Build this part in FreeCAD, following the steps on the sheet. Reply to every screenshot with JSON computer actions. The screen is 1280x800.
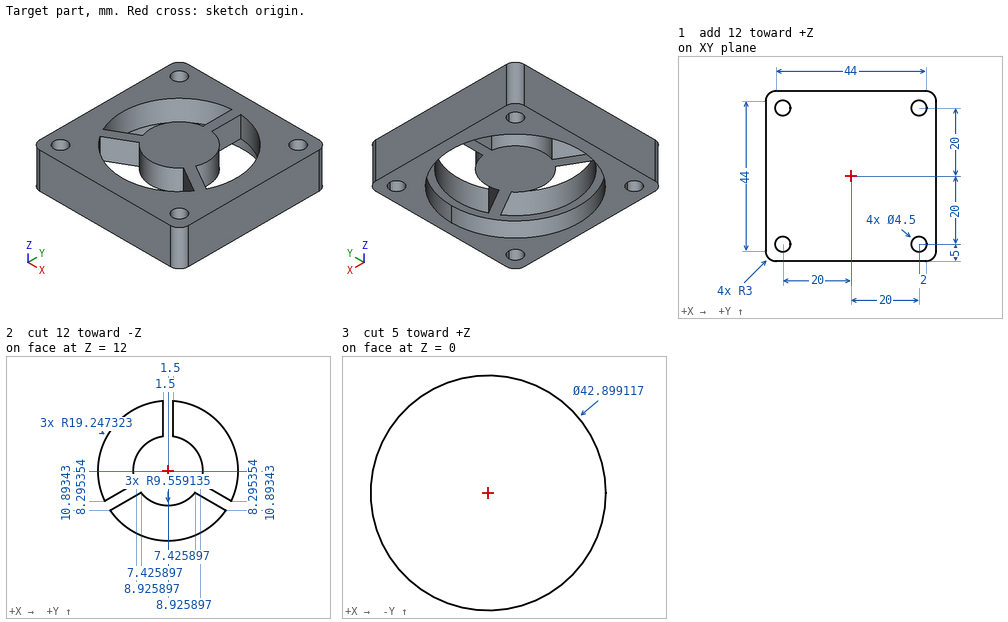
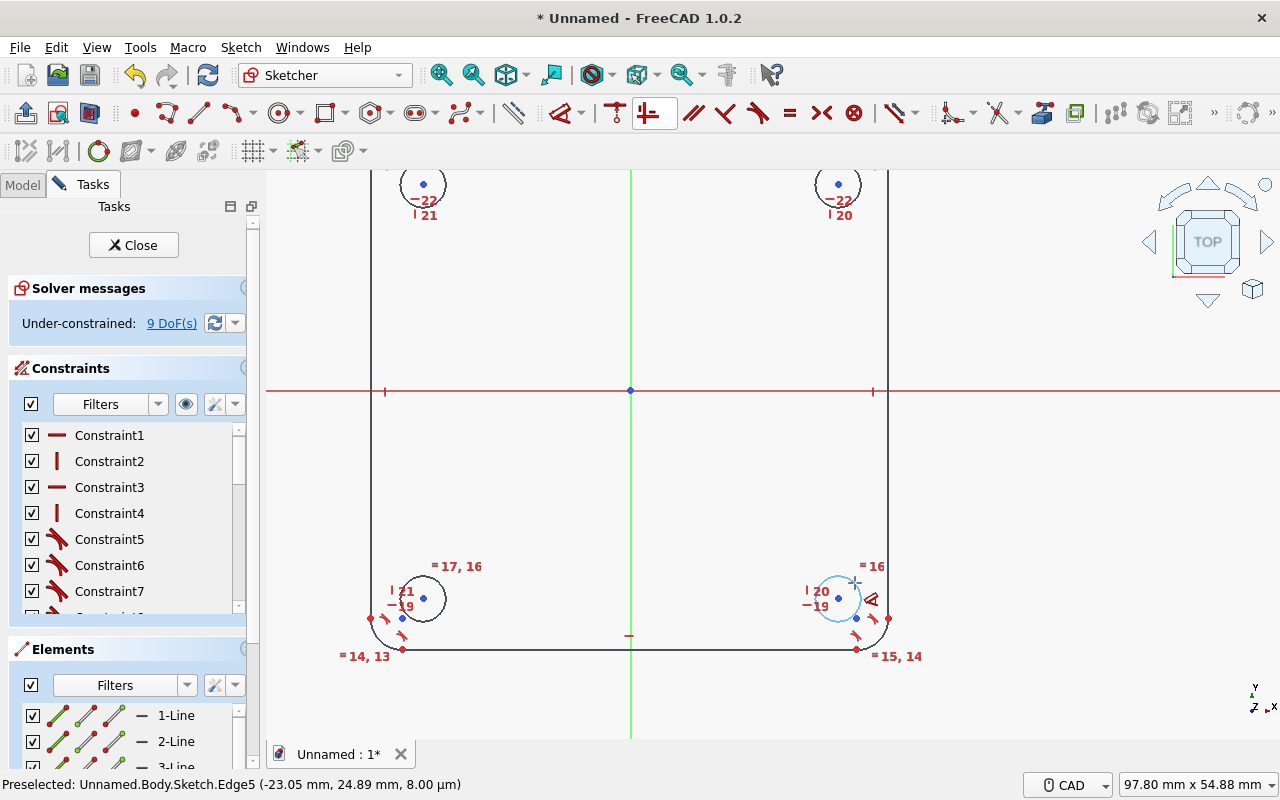
{"action": "left_click", "coordinate": [854, 583]}
{"action": "left_click", "coordinate": [853, 547]}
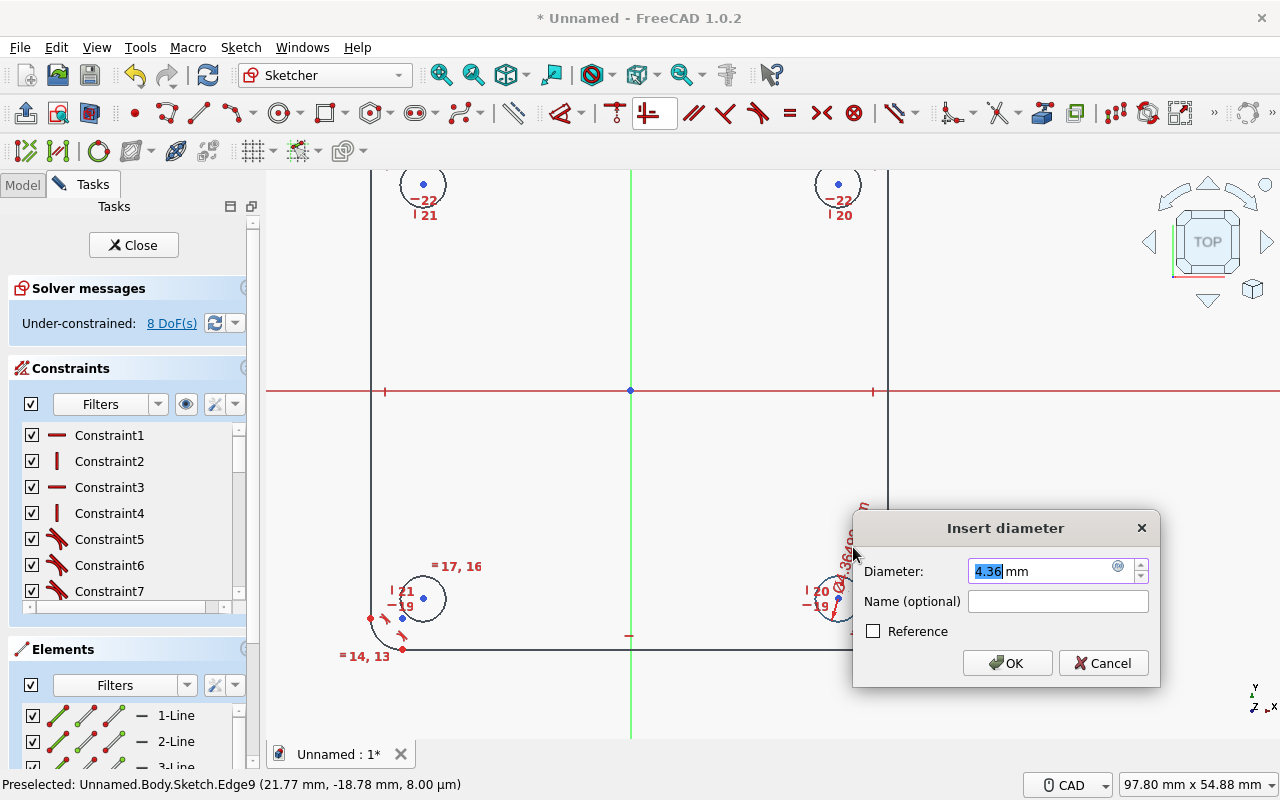
{"action": "type", "text": "4.5"}
{"action": "key", "text": "Return"}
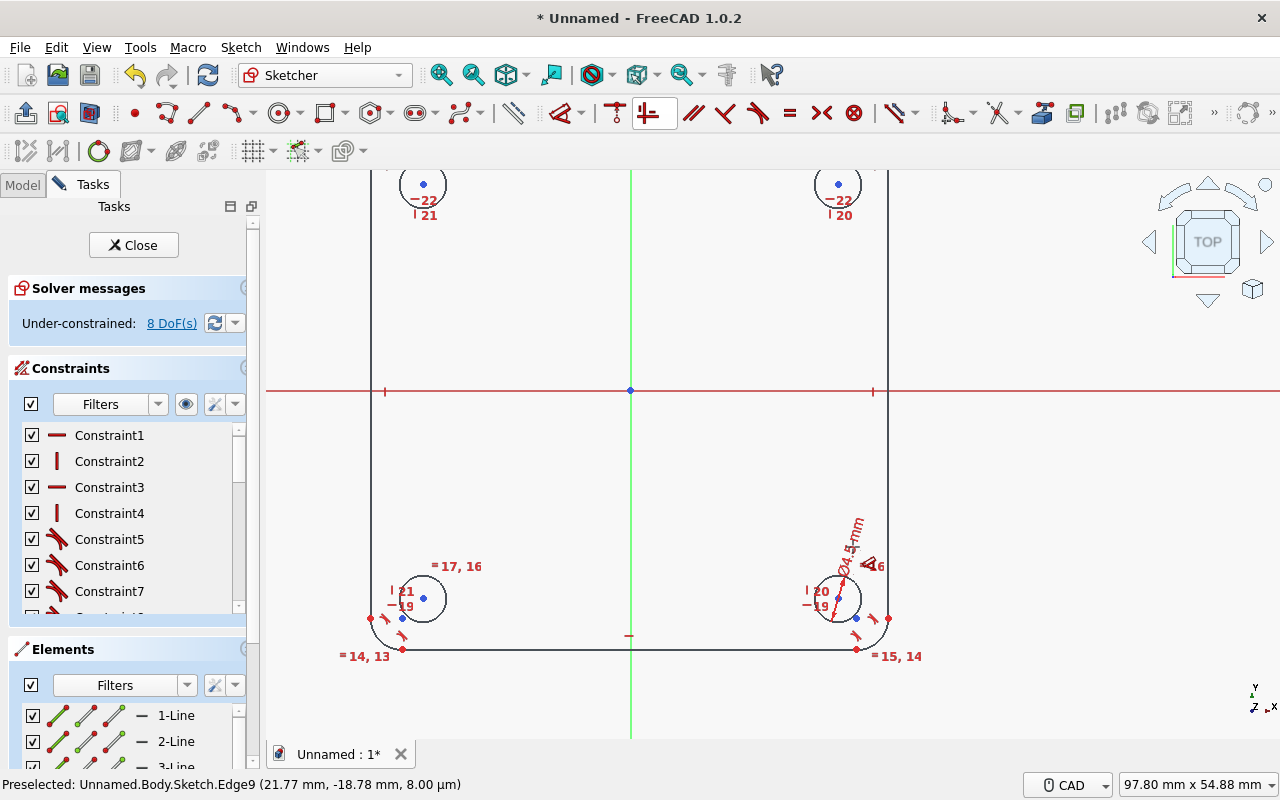
{"action": "scroll", "coordinate": [855, 584], "scroll_direction": "down", "scroll_amount": 2}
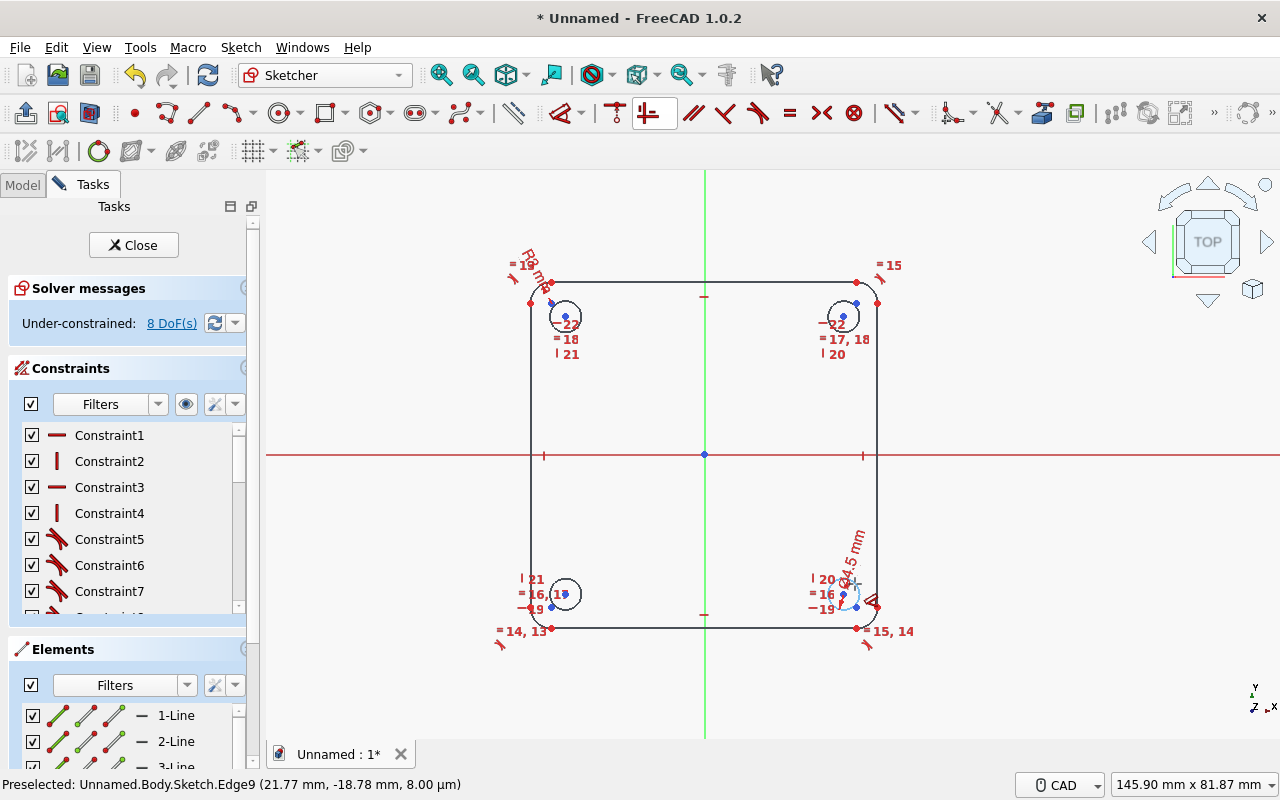
{"action": "left_click", "coordinate": [765, 282]}
{"action": "left_click", "coordinate": [634, 248]}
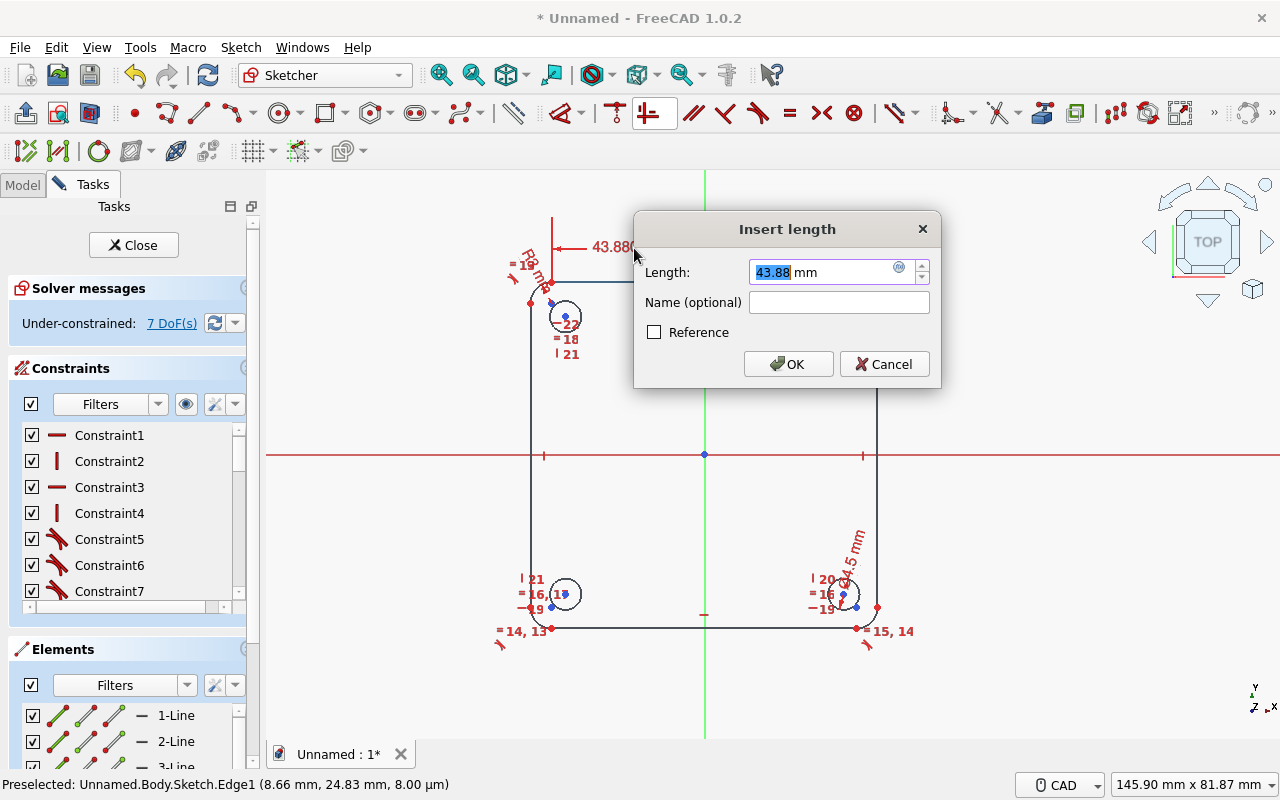
{"action": "type", "text": "44"}
{"action": "key", "text": "Return"}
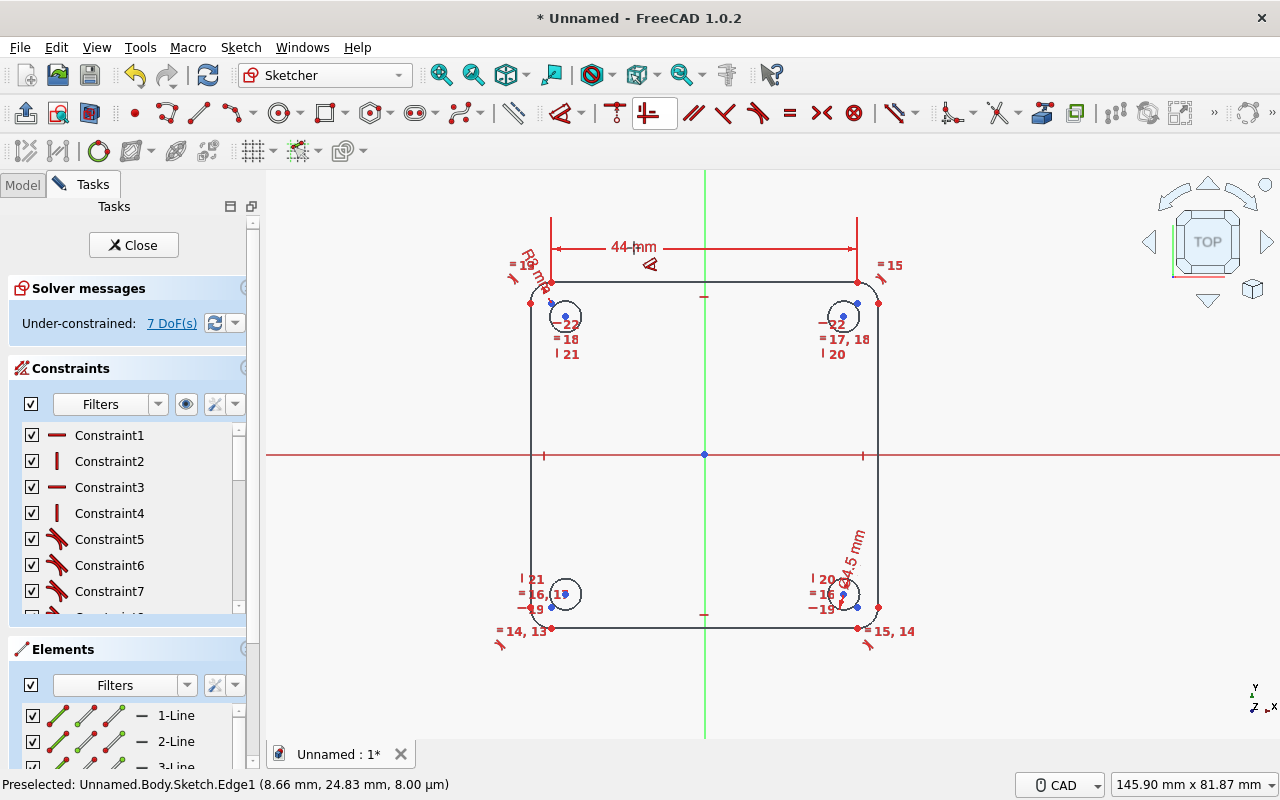
{"action": "left_click", "coordinate": [531, 394]}
{"action": "left_click", "coordinate": [497, 385]}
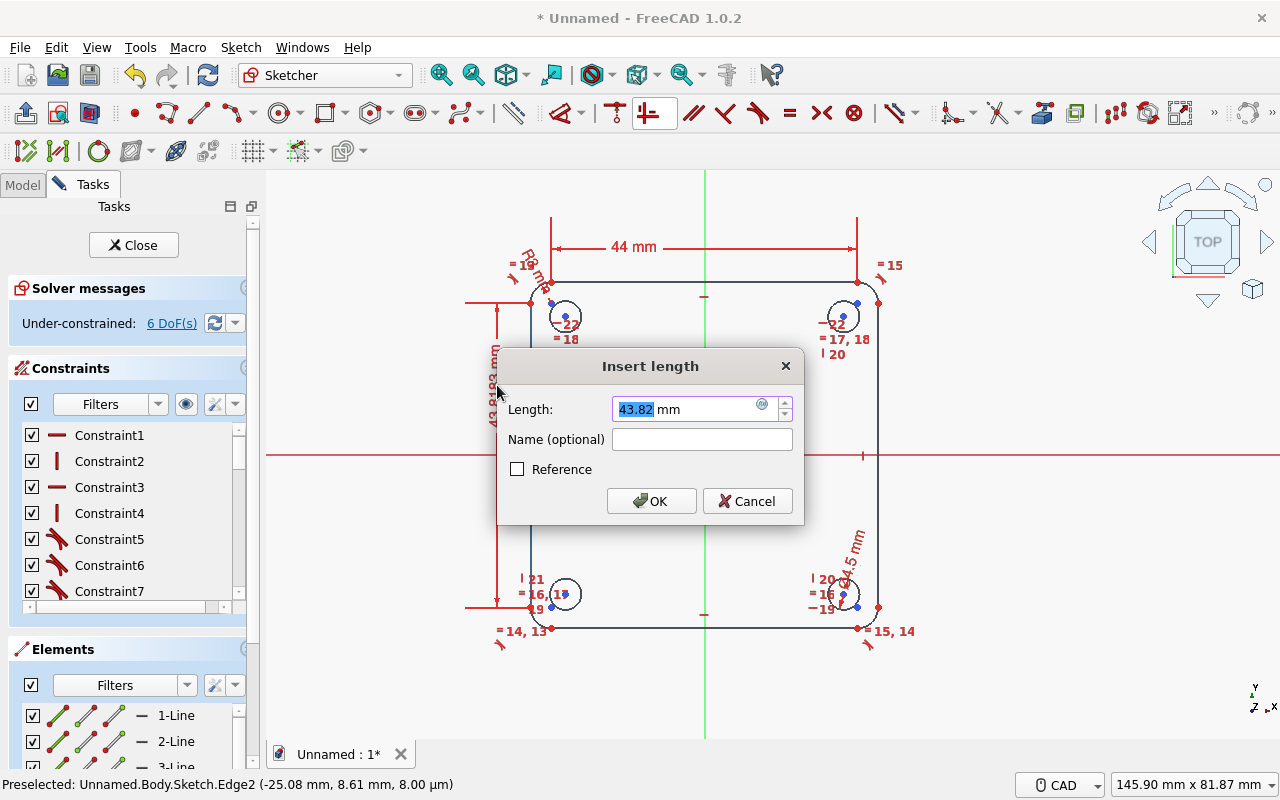
{"action": "type", "text": "44"}
{"action": "key", "text": "Return"}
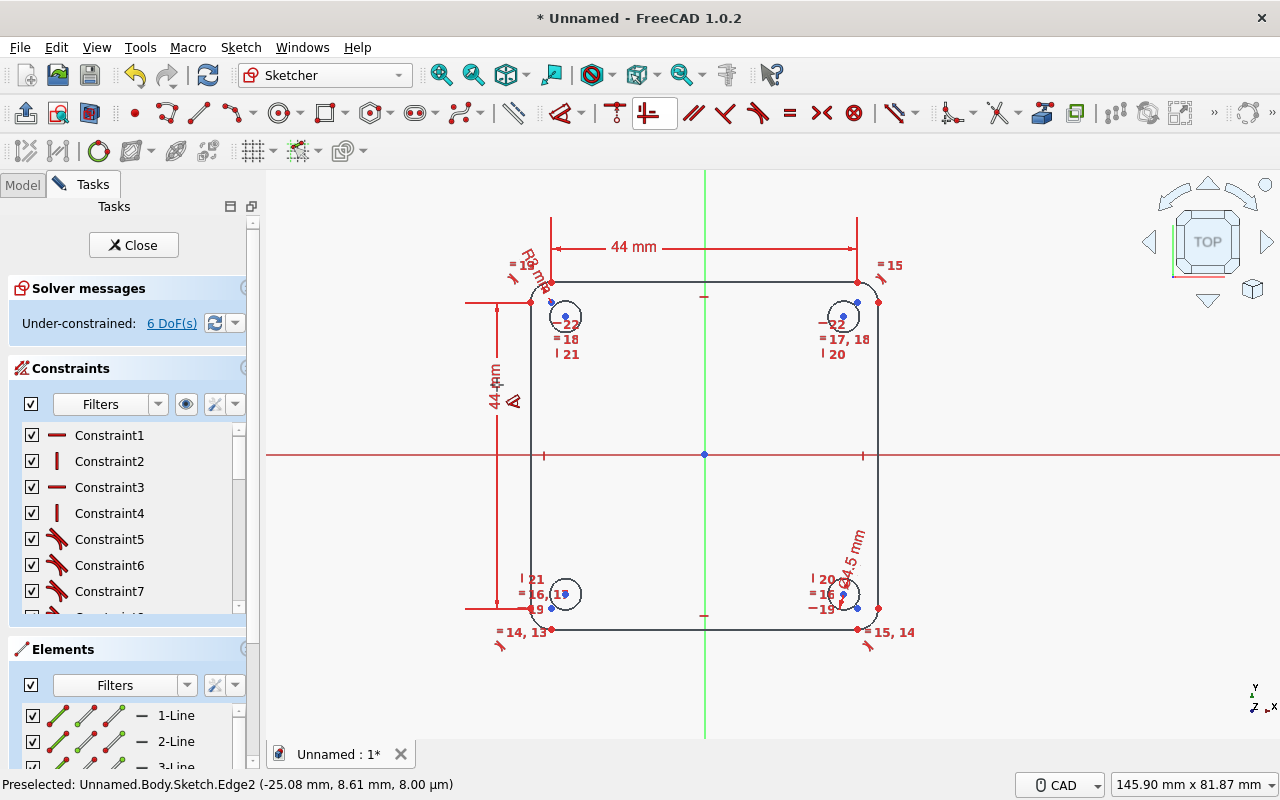
{"action": "left_click", "coordinate": [844, 594]}
{"action": "left_click", "coordinate": [774, 421]}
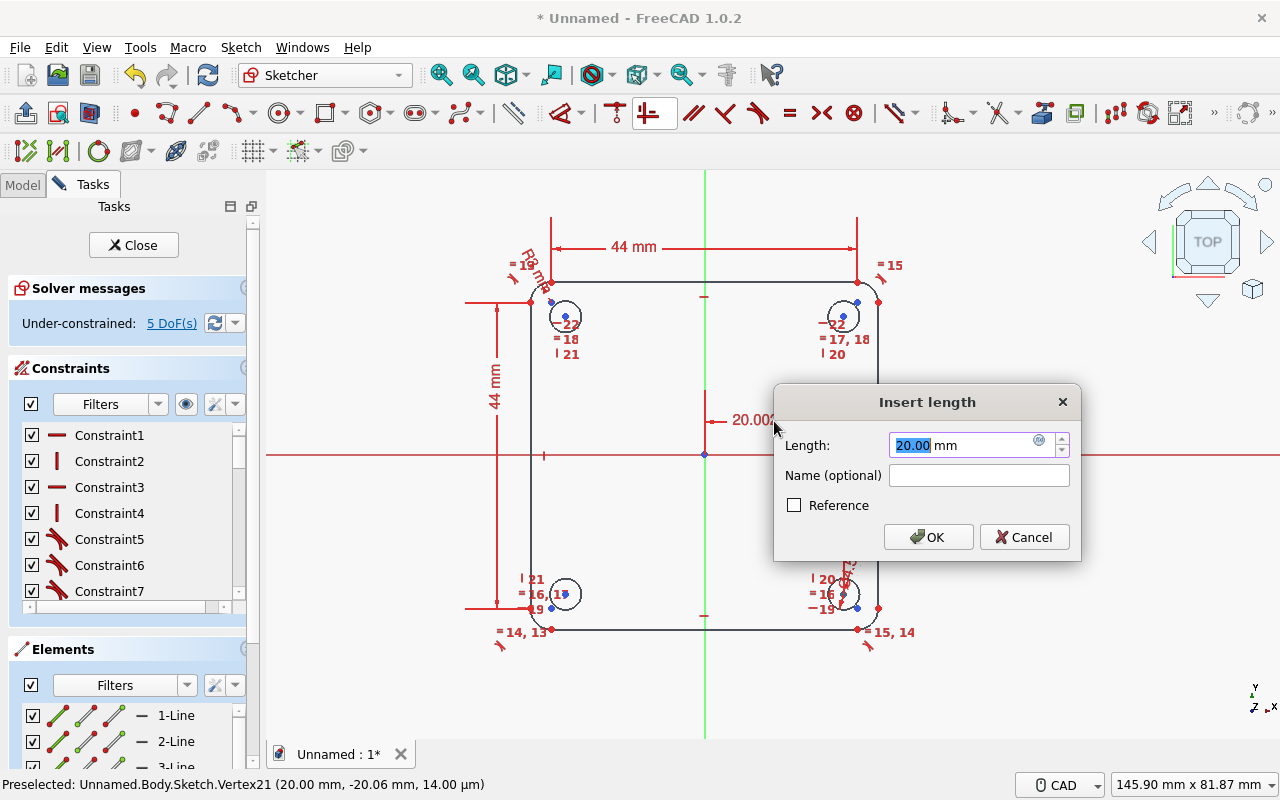
{"action": "type", "text": "20"}
{"action": "key", "text": "Return"}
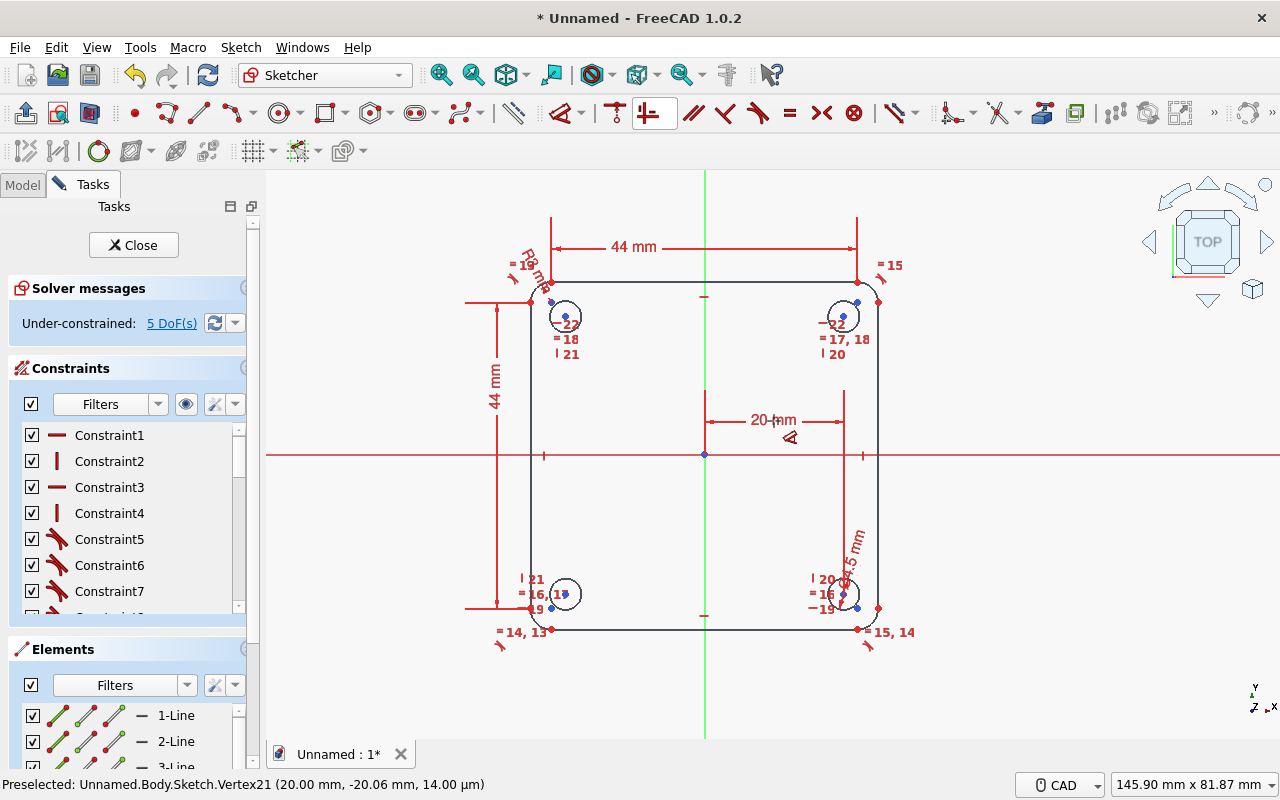
{"action": "left_click", "coordinate": [844, 594]}
{"action": "left_click", "coordinate": [671, 525]}